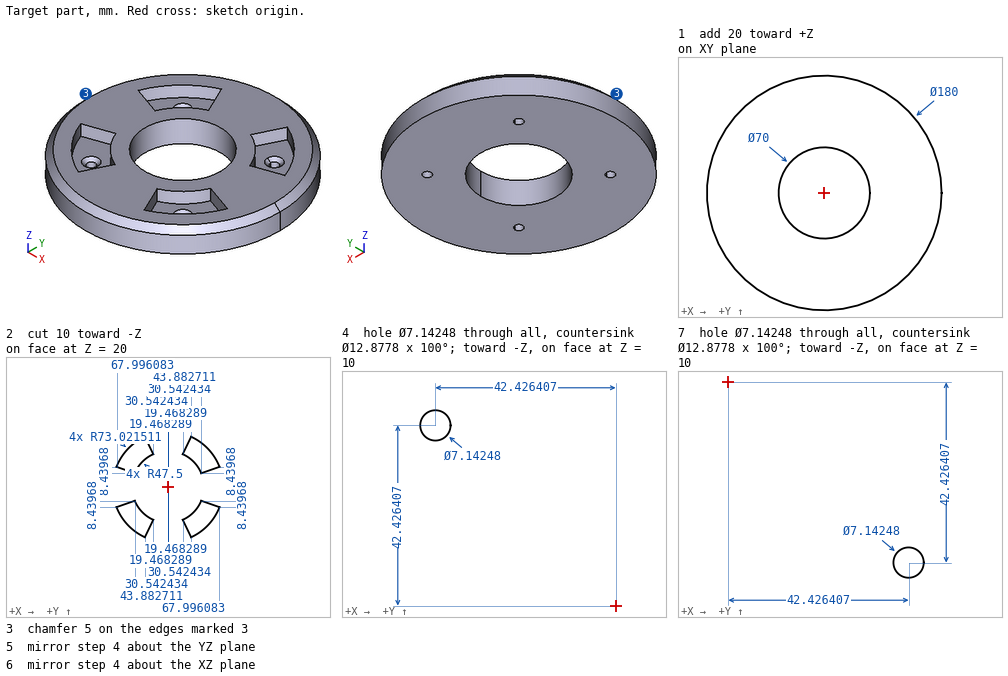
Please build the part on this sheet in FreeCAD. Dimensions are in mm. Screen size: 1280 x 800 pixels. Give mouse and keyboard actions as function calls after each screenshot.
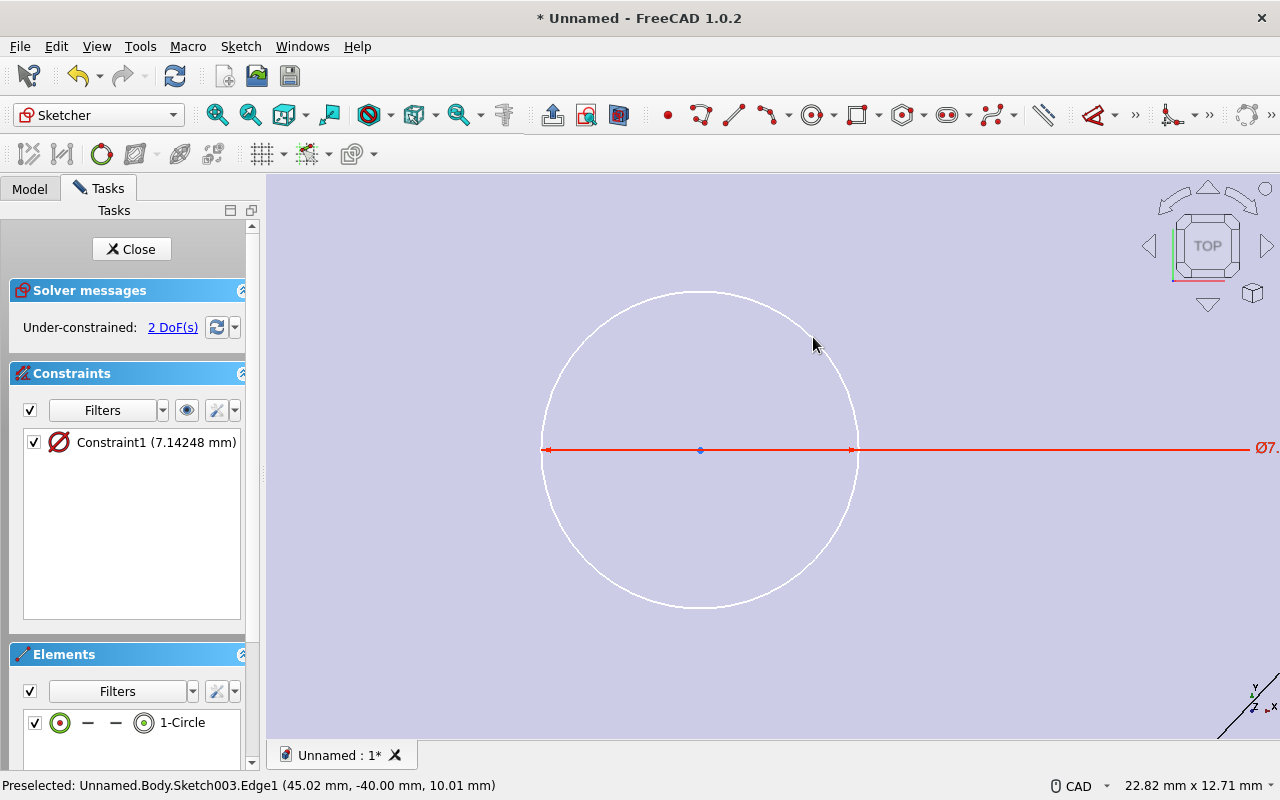
click(1092, 116)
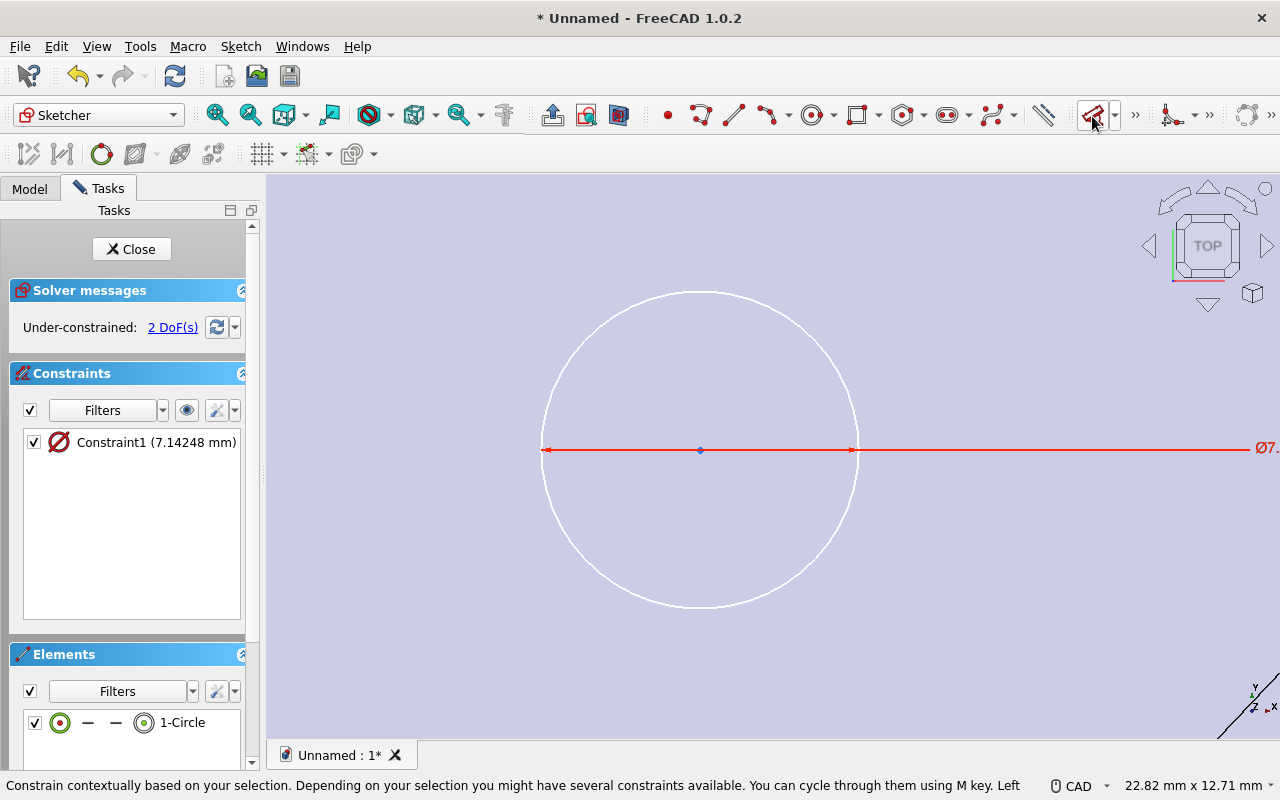
click(700, 450)
click(497, 484)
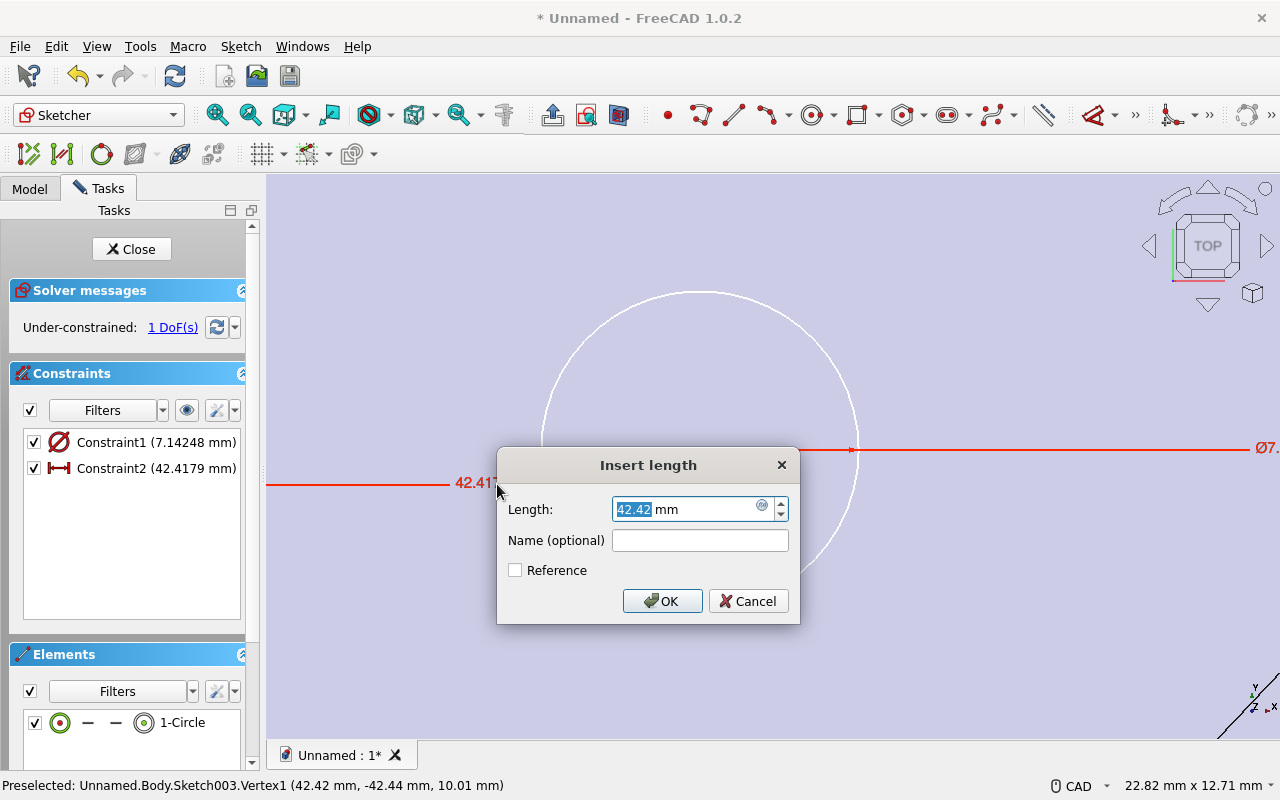
text(42.426407)
key(Return)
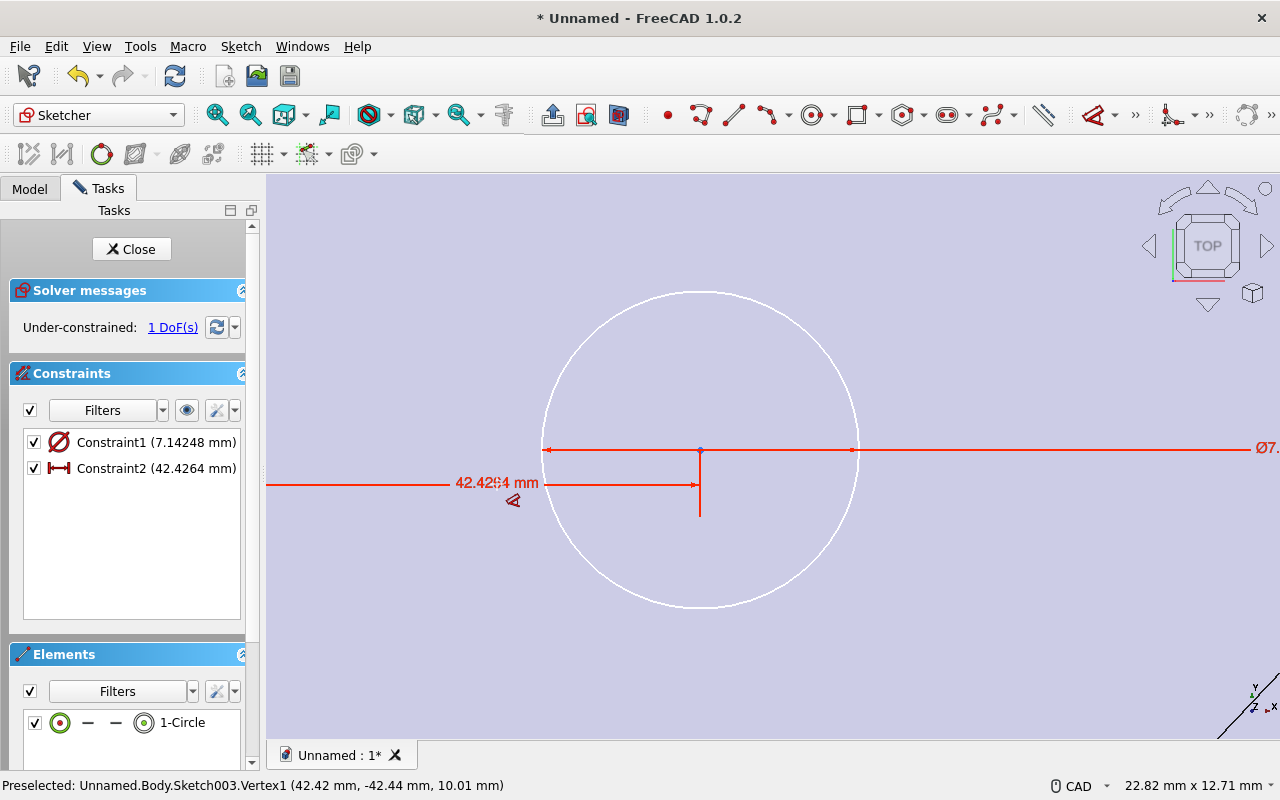
click(700, 450)
click(734, 326)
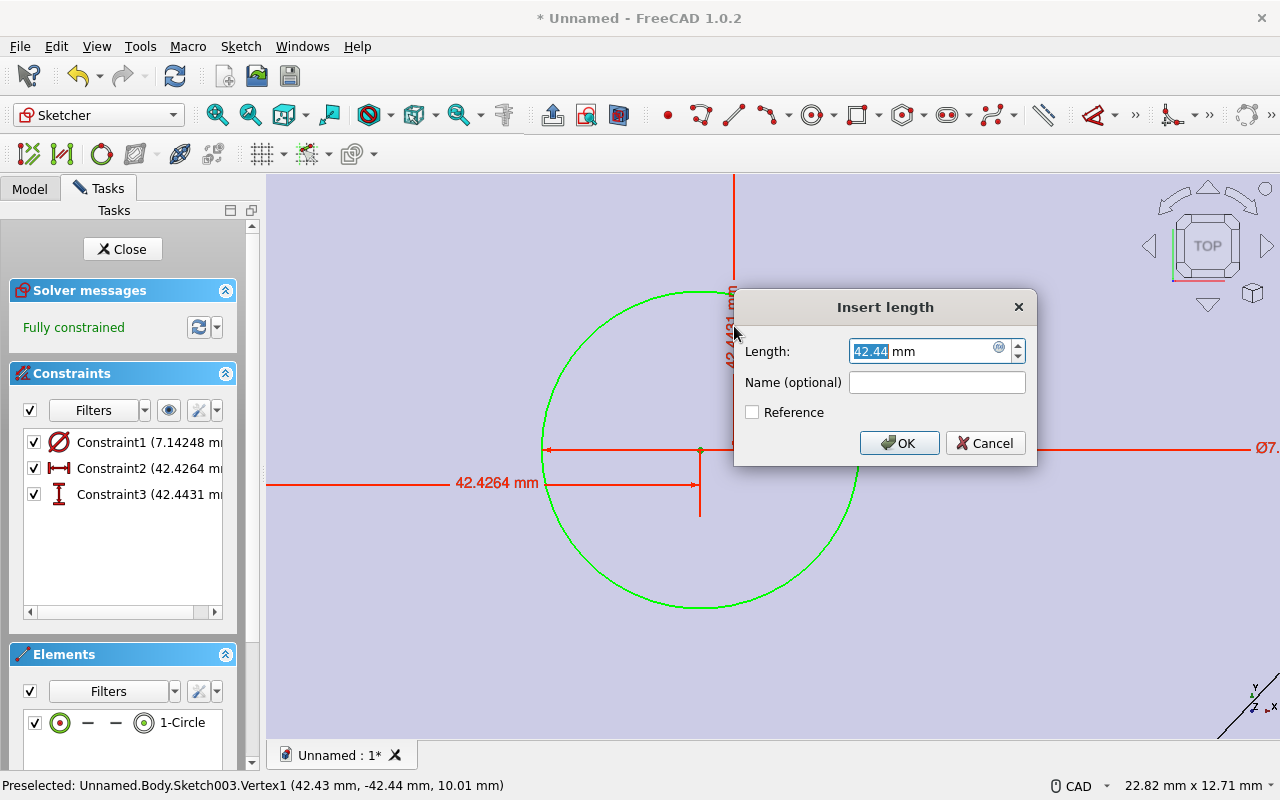
text(42.426407)
key(Return)
key(Escape)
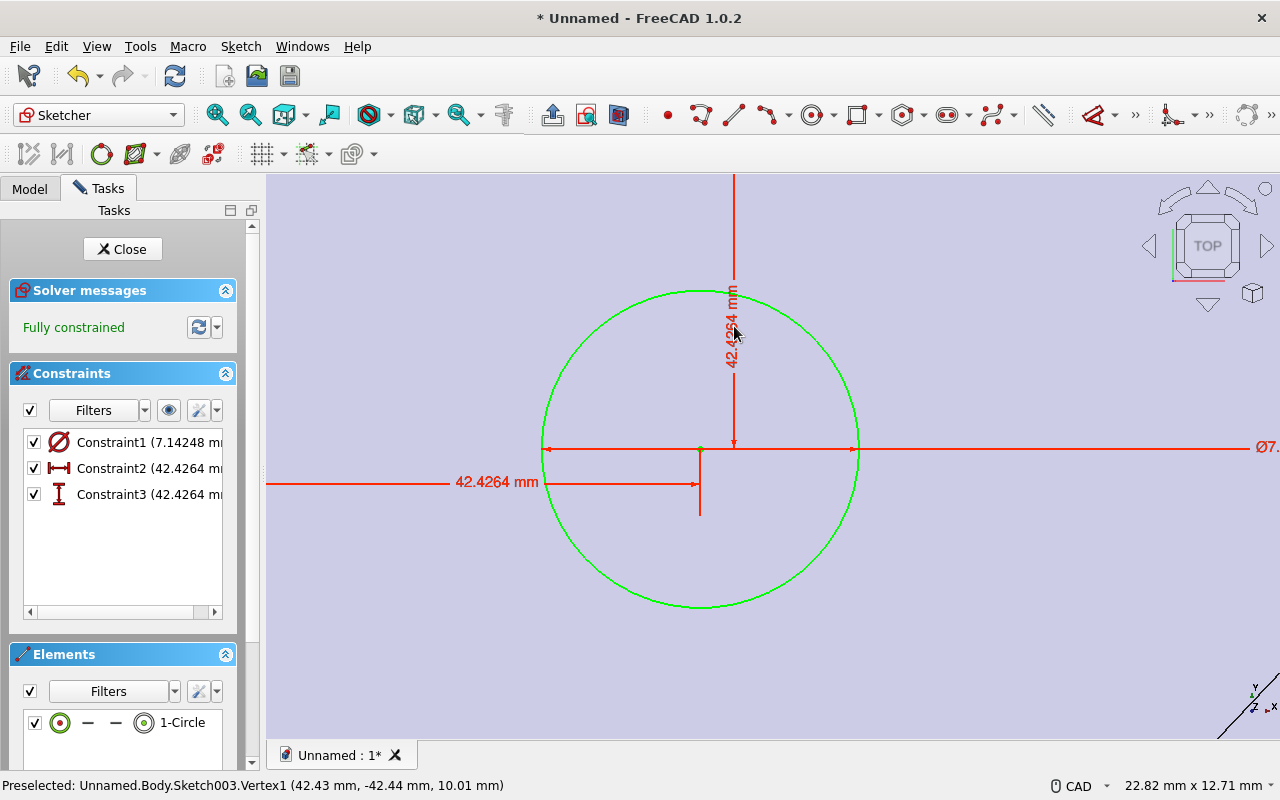
click(123, 249)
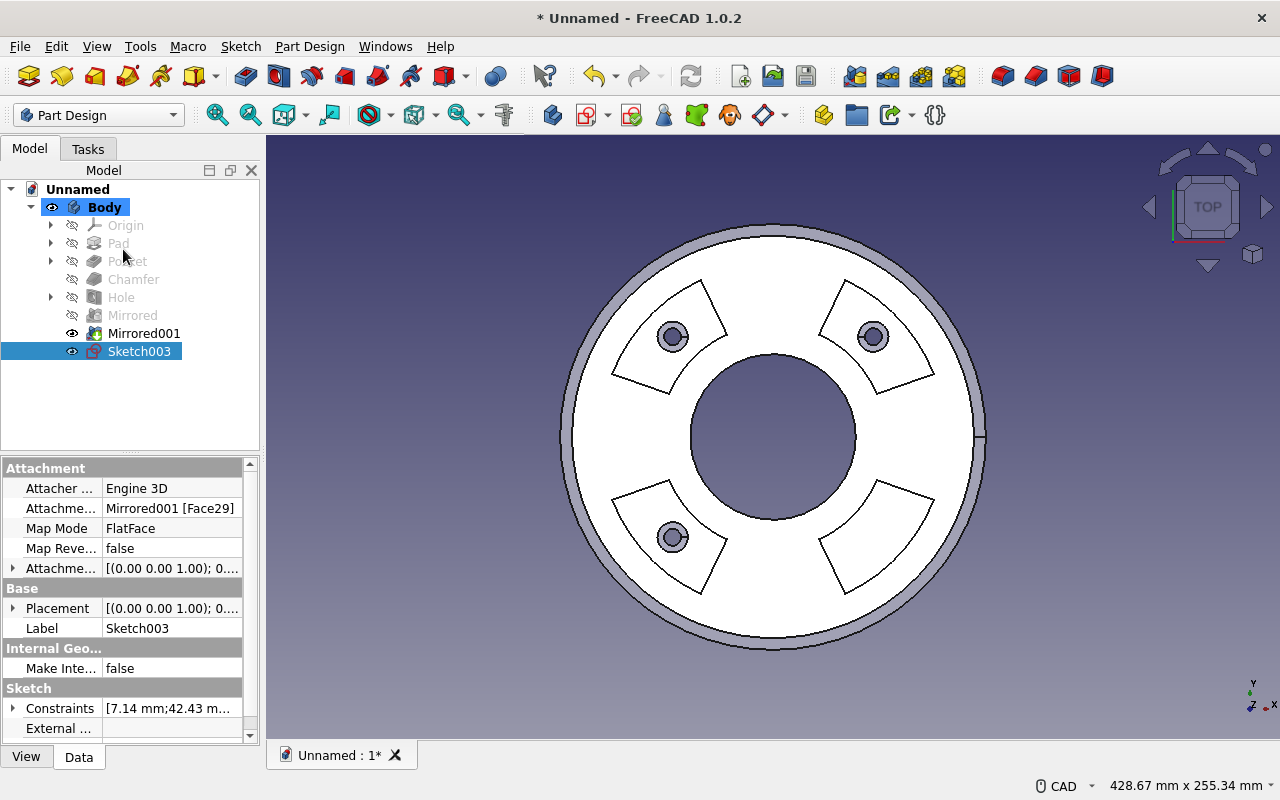
click(279, 76)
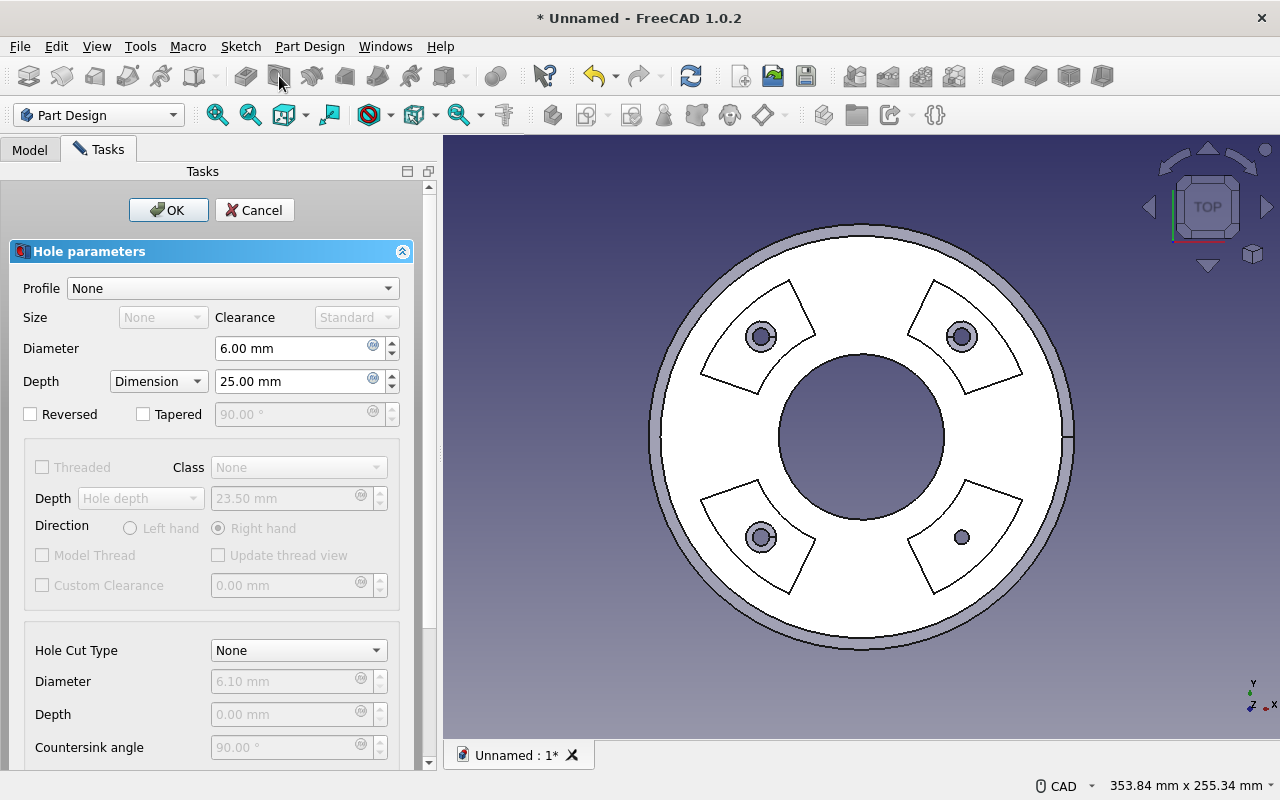
triple_click(300, 348)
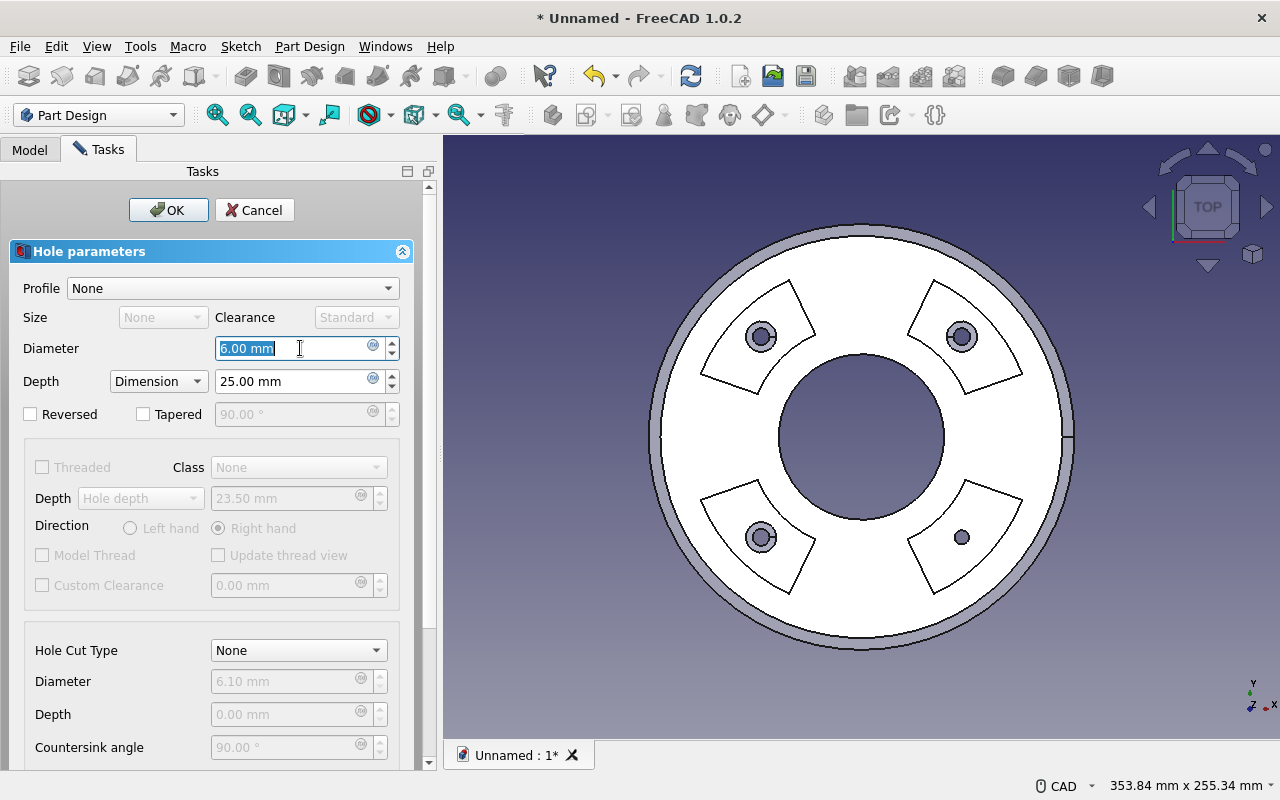
text(7.14248)
key(Tab)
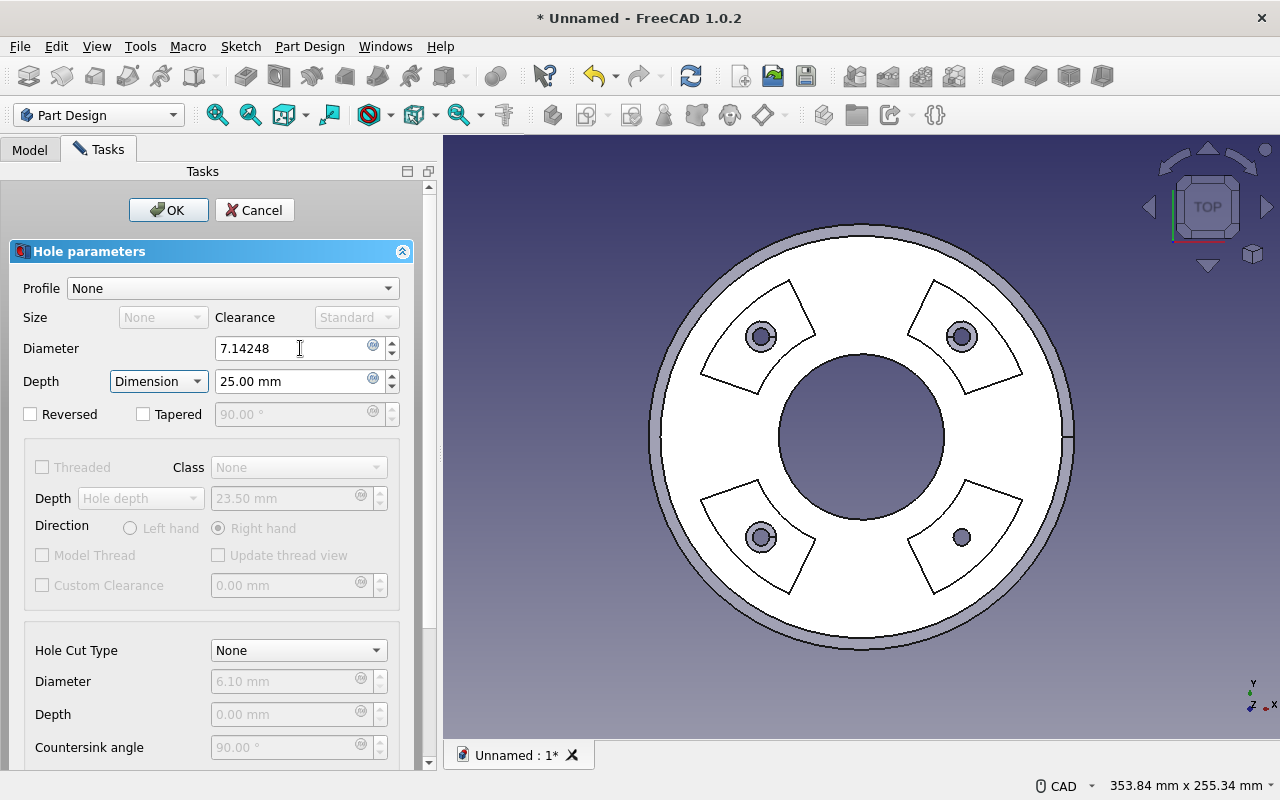
click(160, 382)